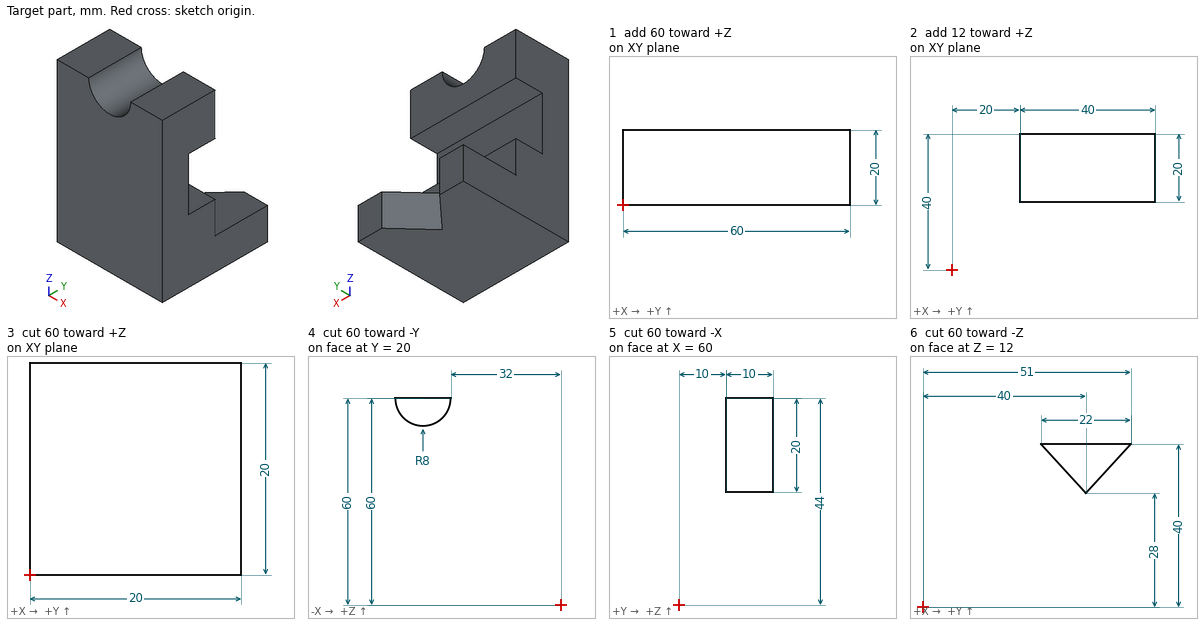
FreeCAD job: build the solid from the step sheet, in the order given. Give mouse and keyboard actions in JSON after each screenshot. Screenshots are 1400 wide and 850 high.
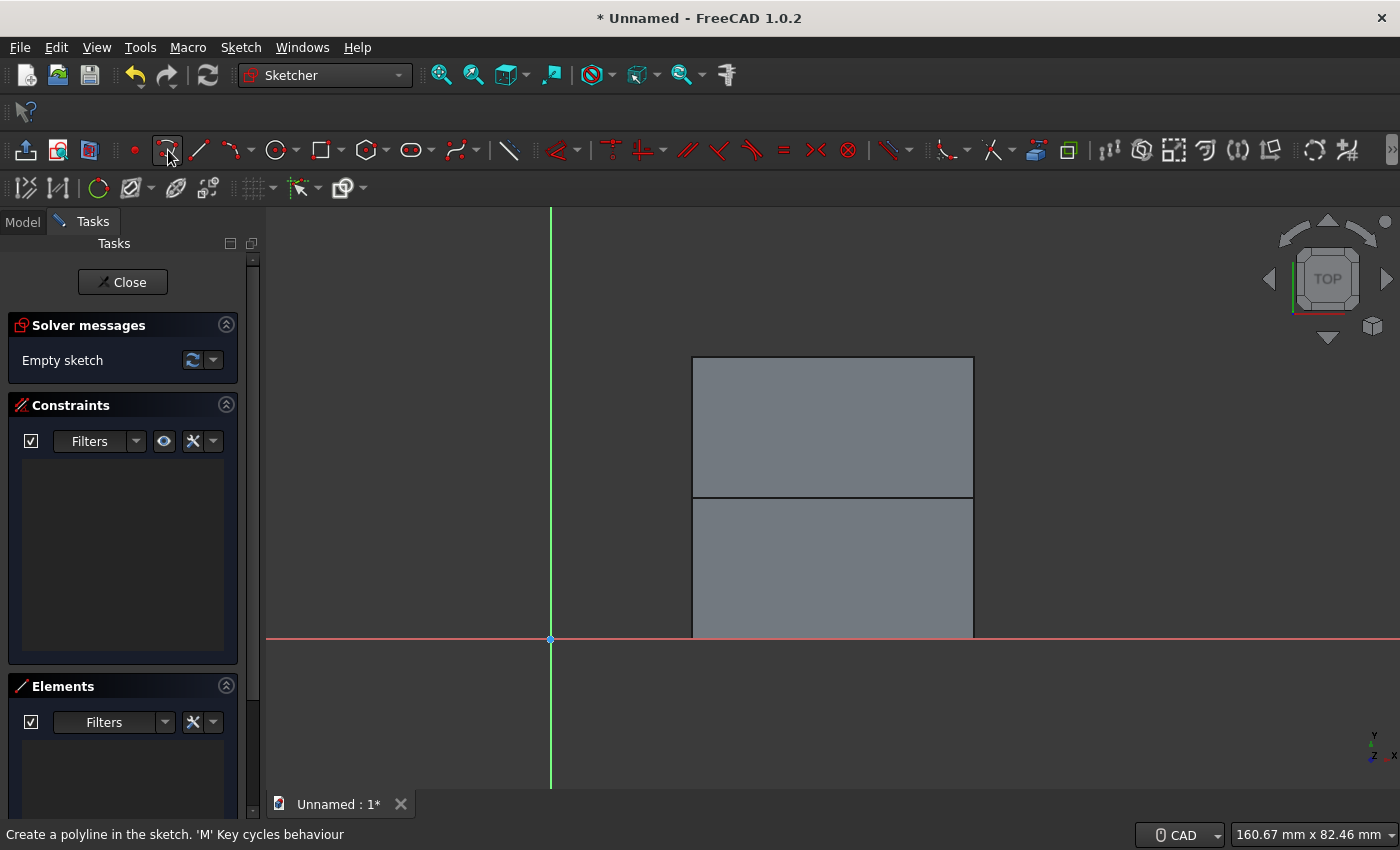
{"action": "left_click", "coordinate": [833, 442]}
{"action": "left_click", "coordinate": [911, 357]}
{"action": "left_click", "coordinate": [755, 357]}
{"action": "left_click", "coordinate": [833, 443]}
{"action": "key", "text": "Escape"}
{"action": "key", "text": "Escape"}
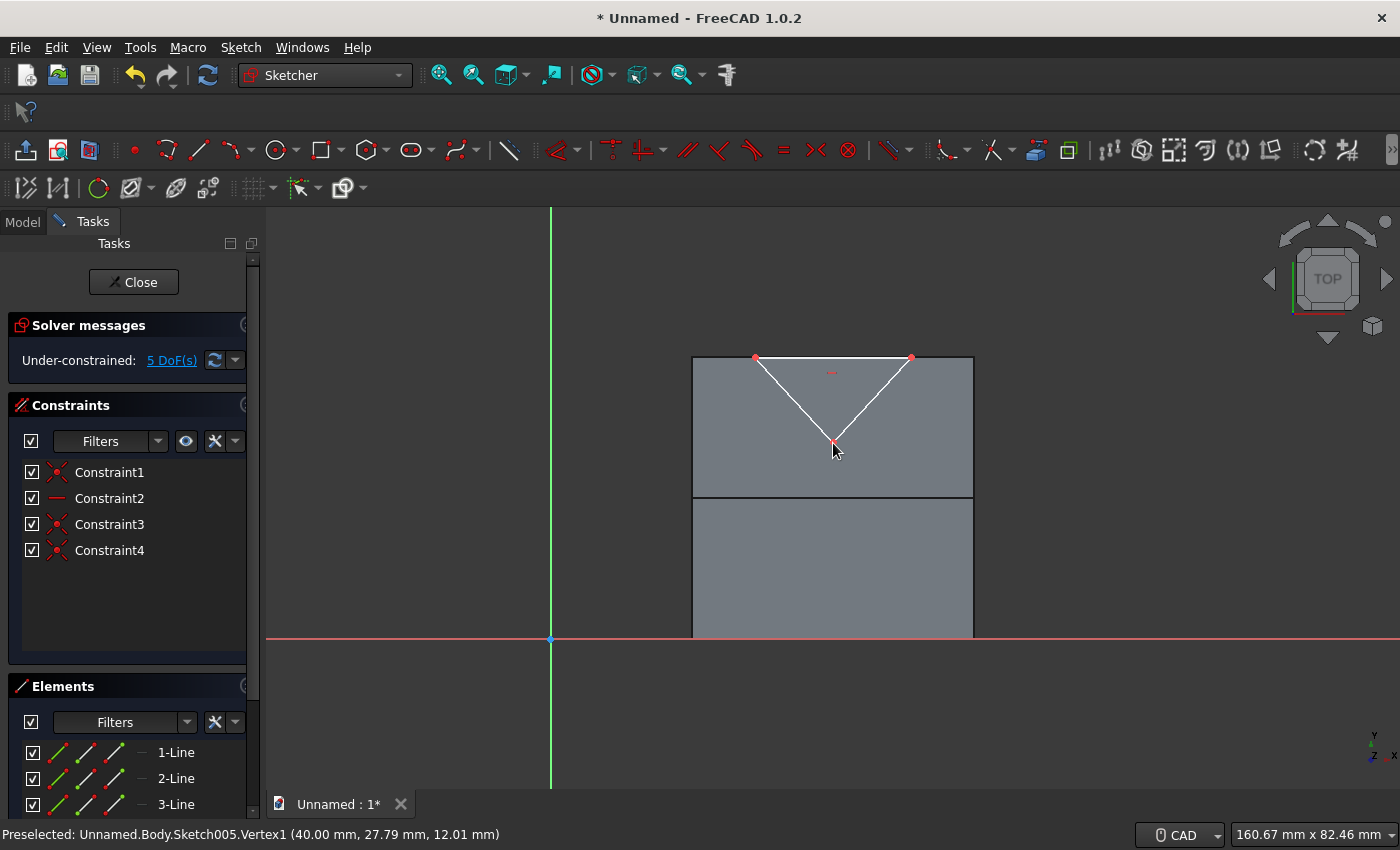
{"action": "left_click", "coordinate": [556, 150]}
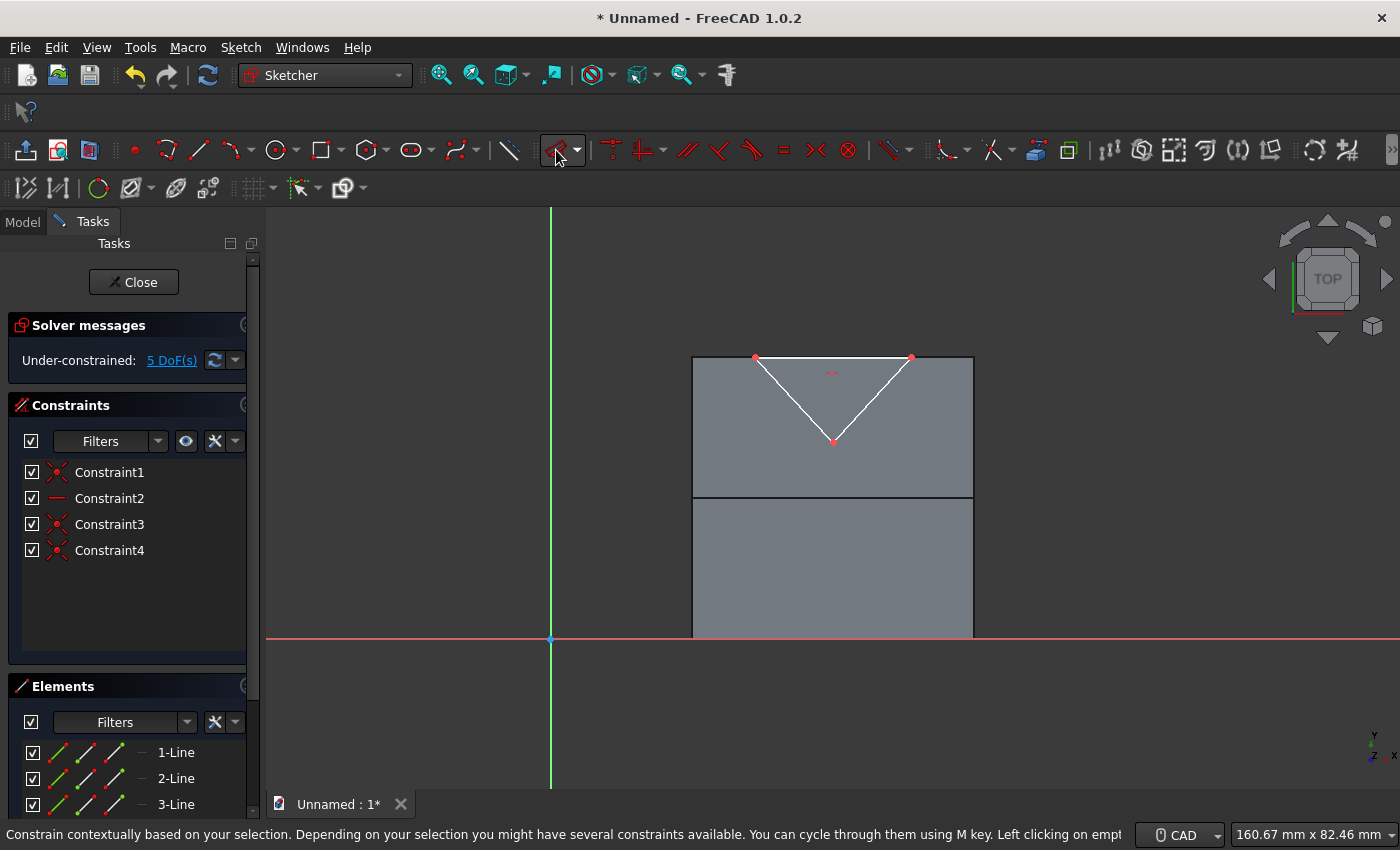
{"action": "left_click", "coordinate": [864, 358]}
{"action": "left_click", "coordinate": [833, 324]}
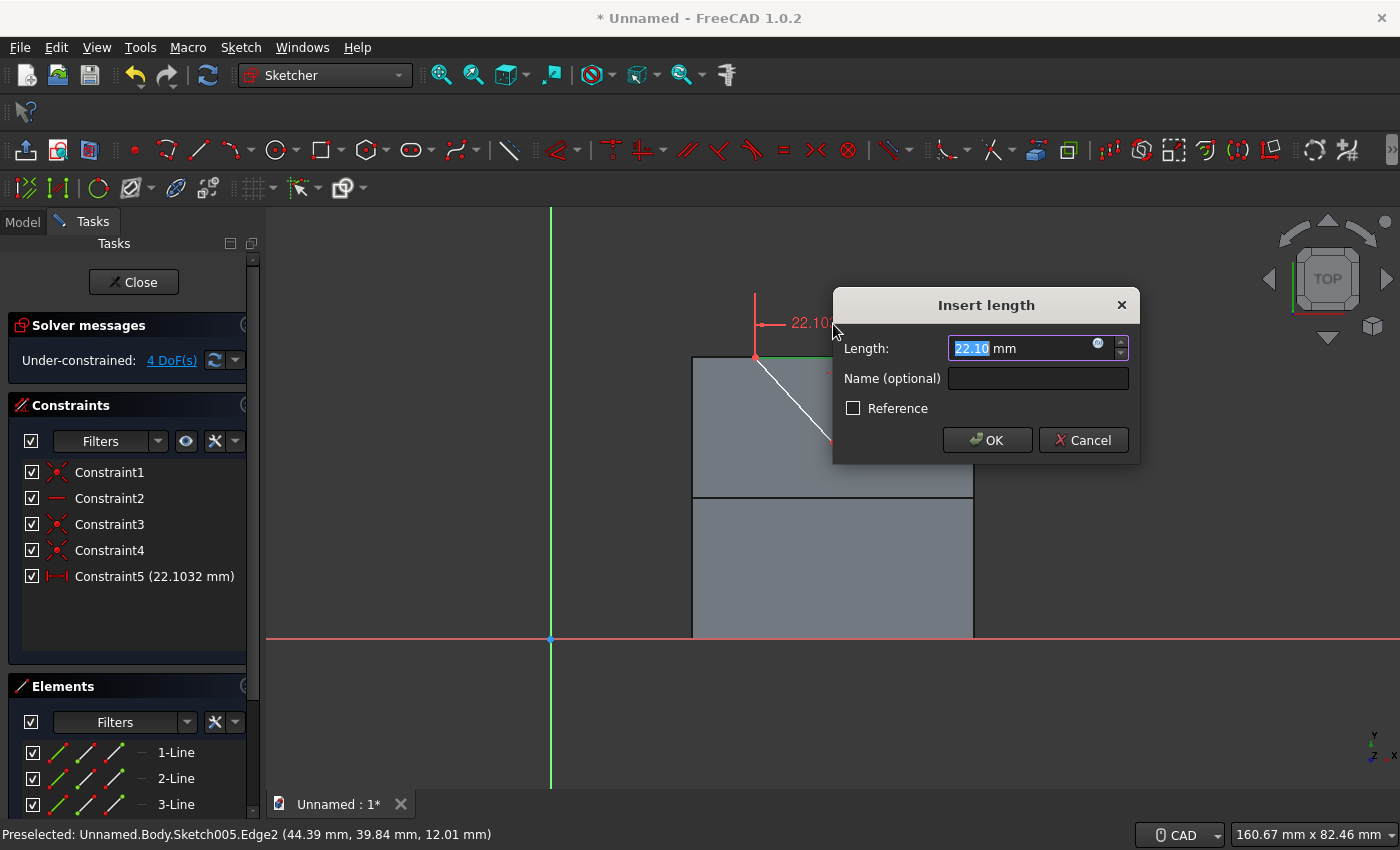
{"action": "type", "text": "22"}
{"action": "key", "text": "Return"}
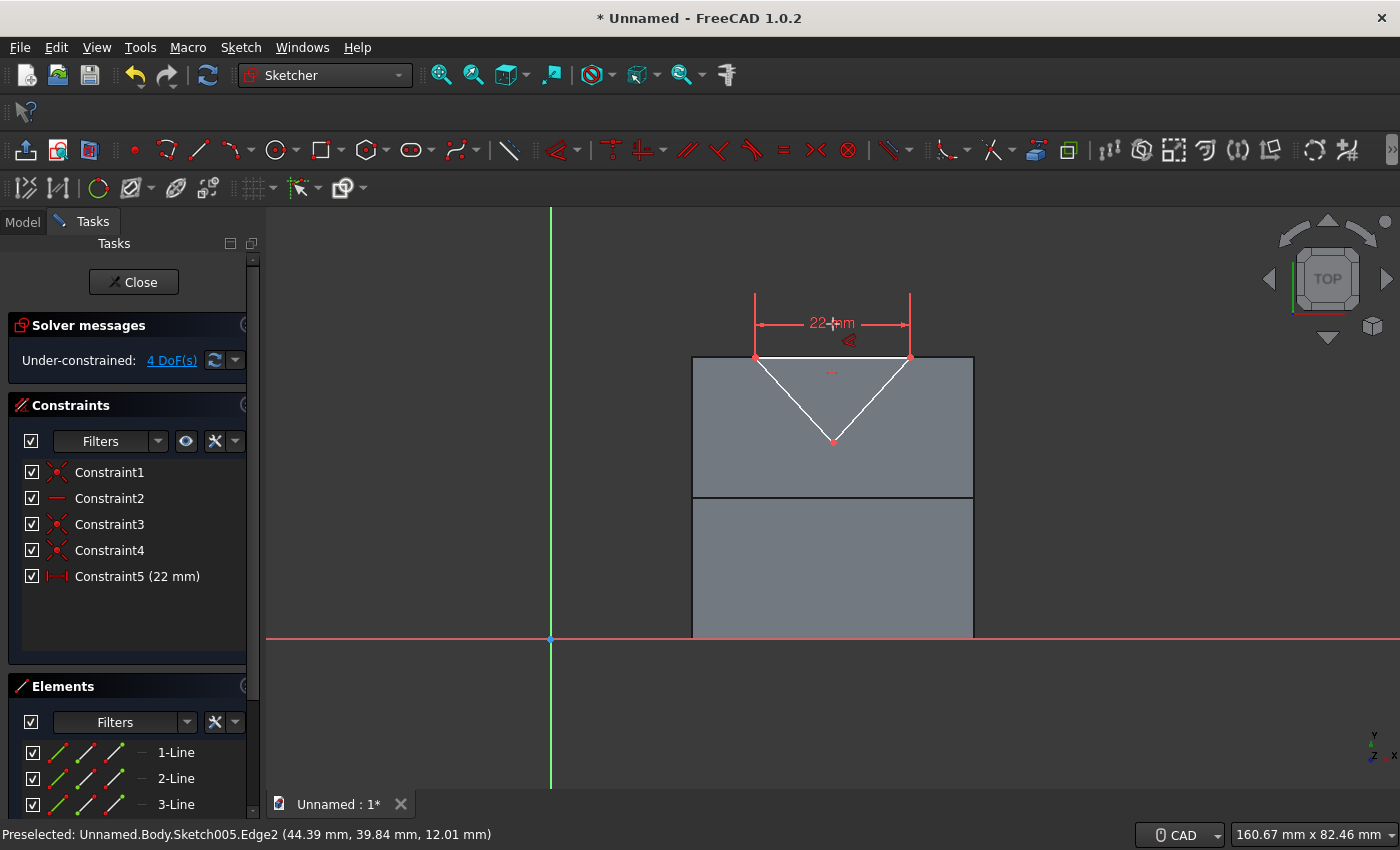
{"action": "left_click", "coordinate": [833, 443]}
{"action": "left_click", "coordinate": [692, 673]}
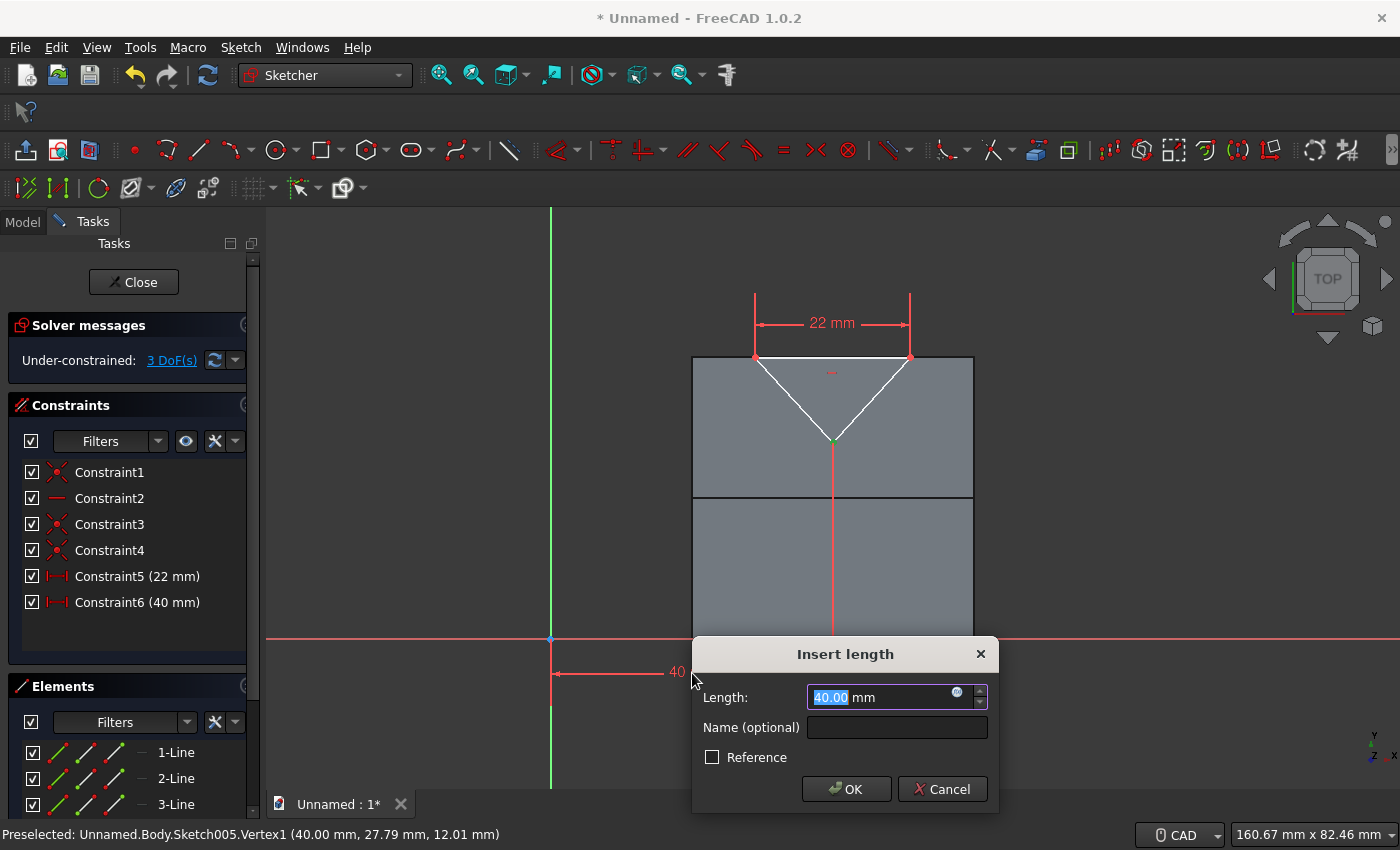
{"action": "type", "text": "40"}
{"action": "key", "text": "Return"}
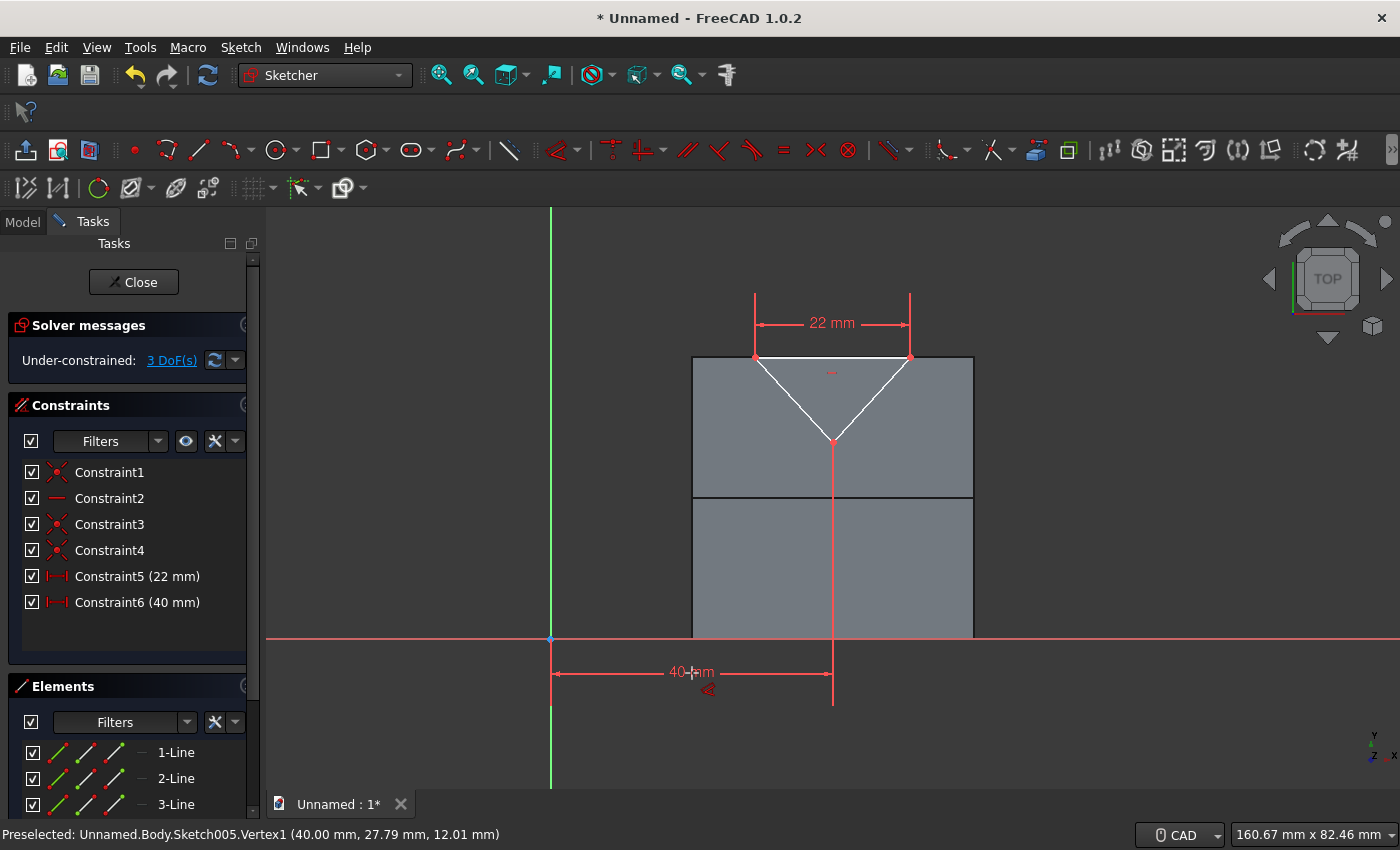
{"action": "left_click", "coordinate": [833, 443]}
{"action": "left_click", "coordinate": [517, 541]}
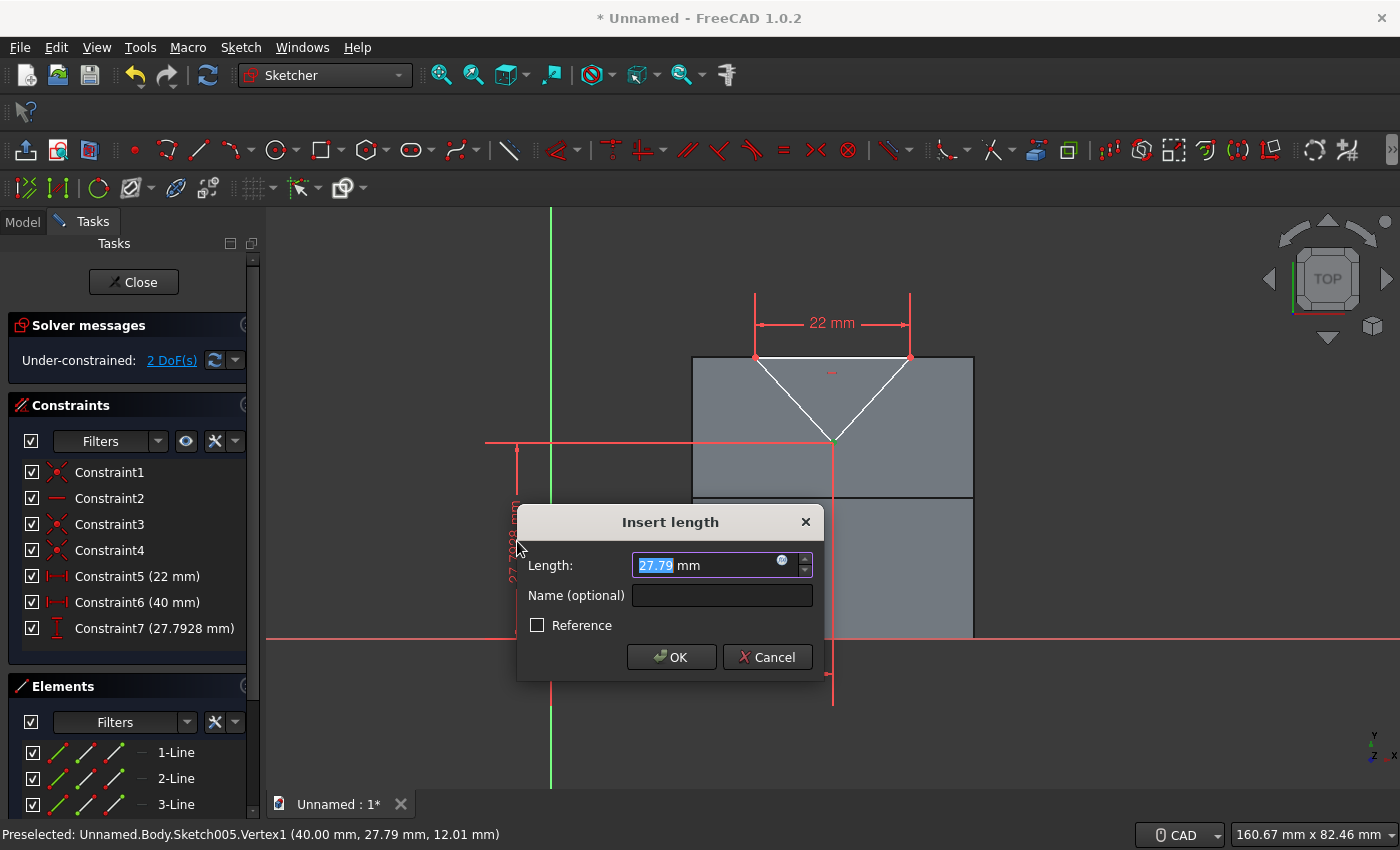
{"action": "type", "text": "28"}
{"action": "key", "text": "Return"}